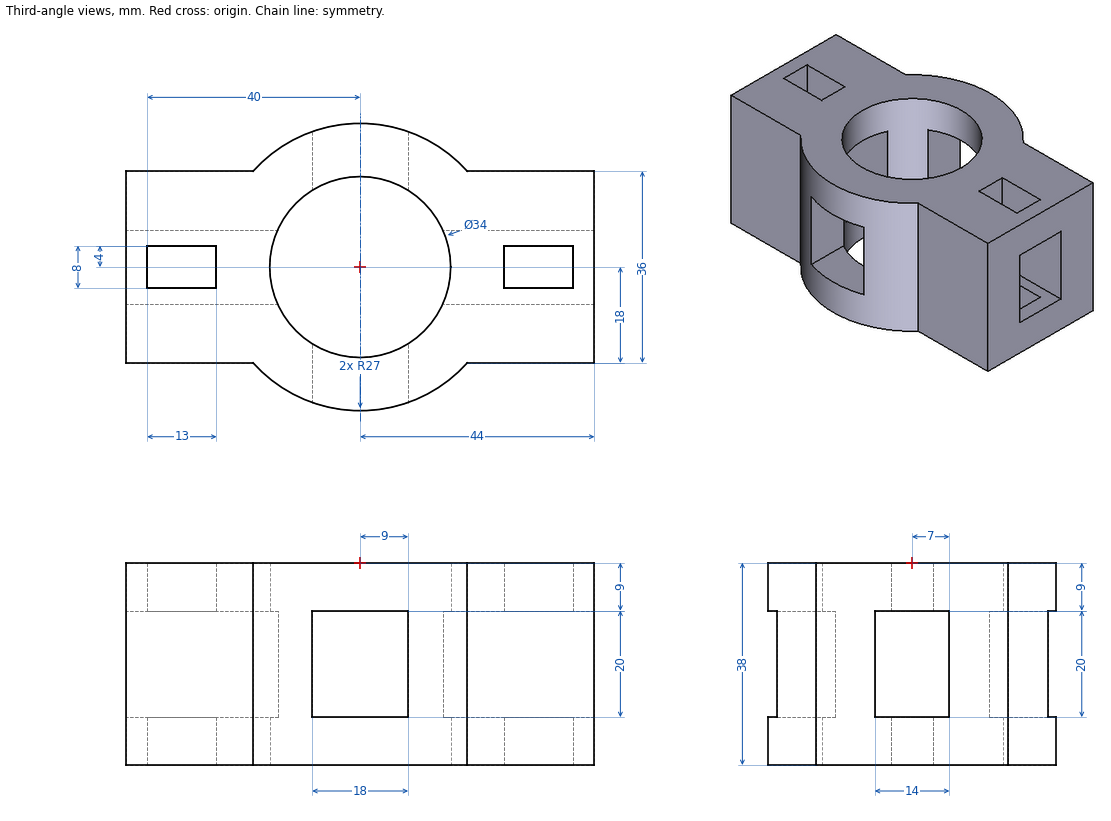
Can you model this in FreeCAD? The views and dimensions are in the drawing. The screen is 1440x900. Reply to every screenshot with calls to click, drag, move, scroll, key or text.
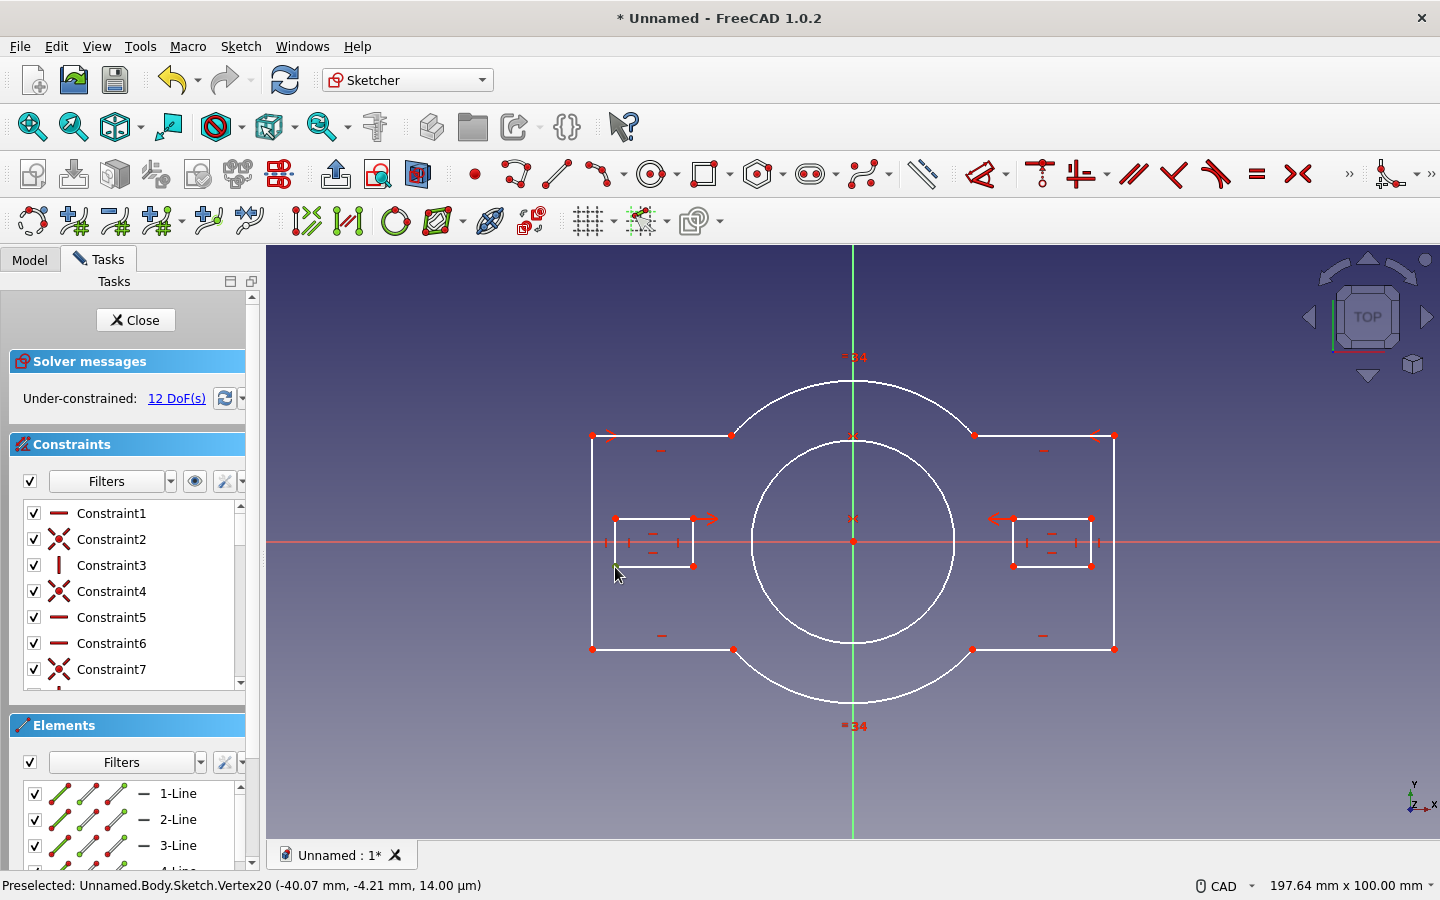
click(1091, 567)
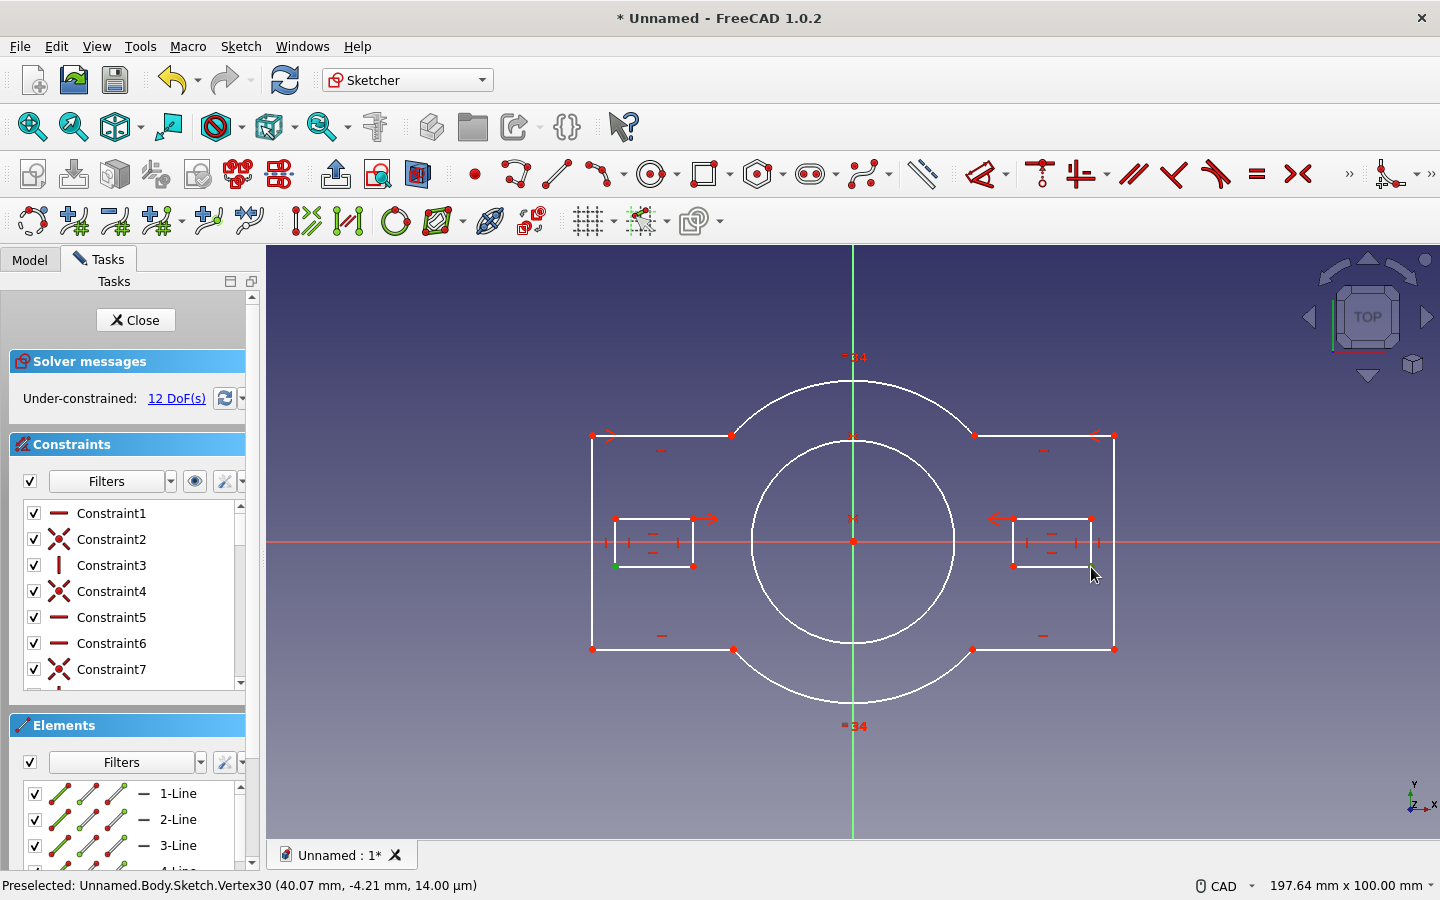
click(853, 773)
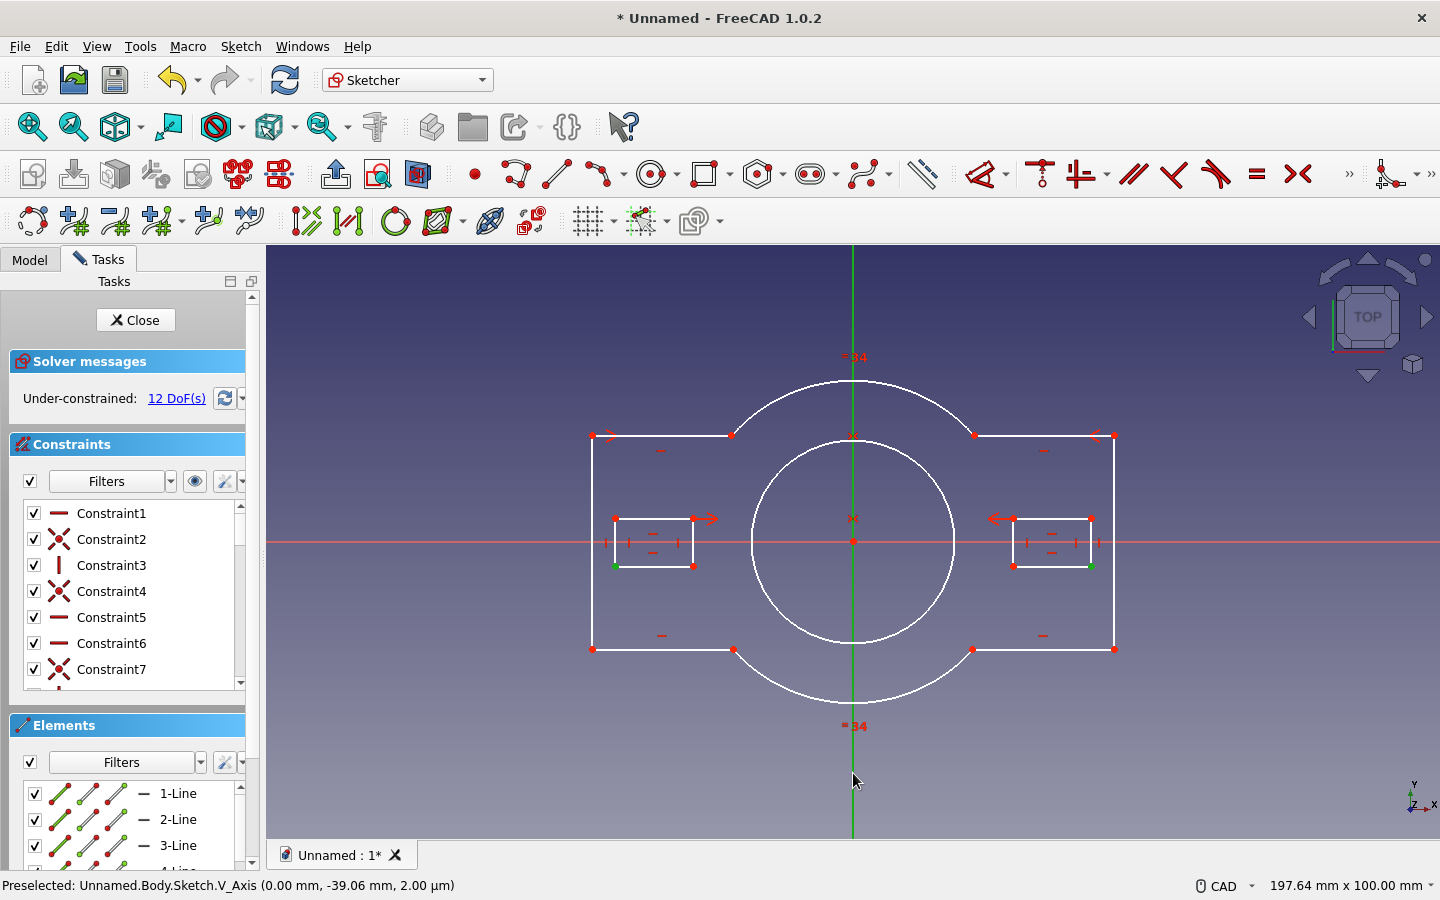
click(1298, 174)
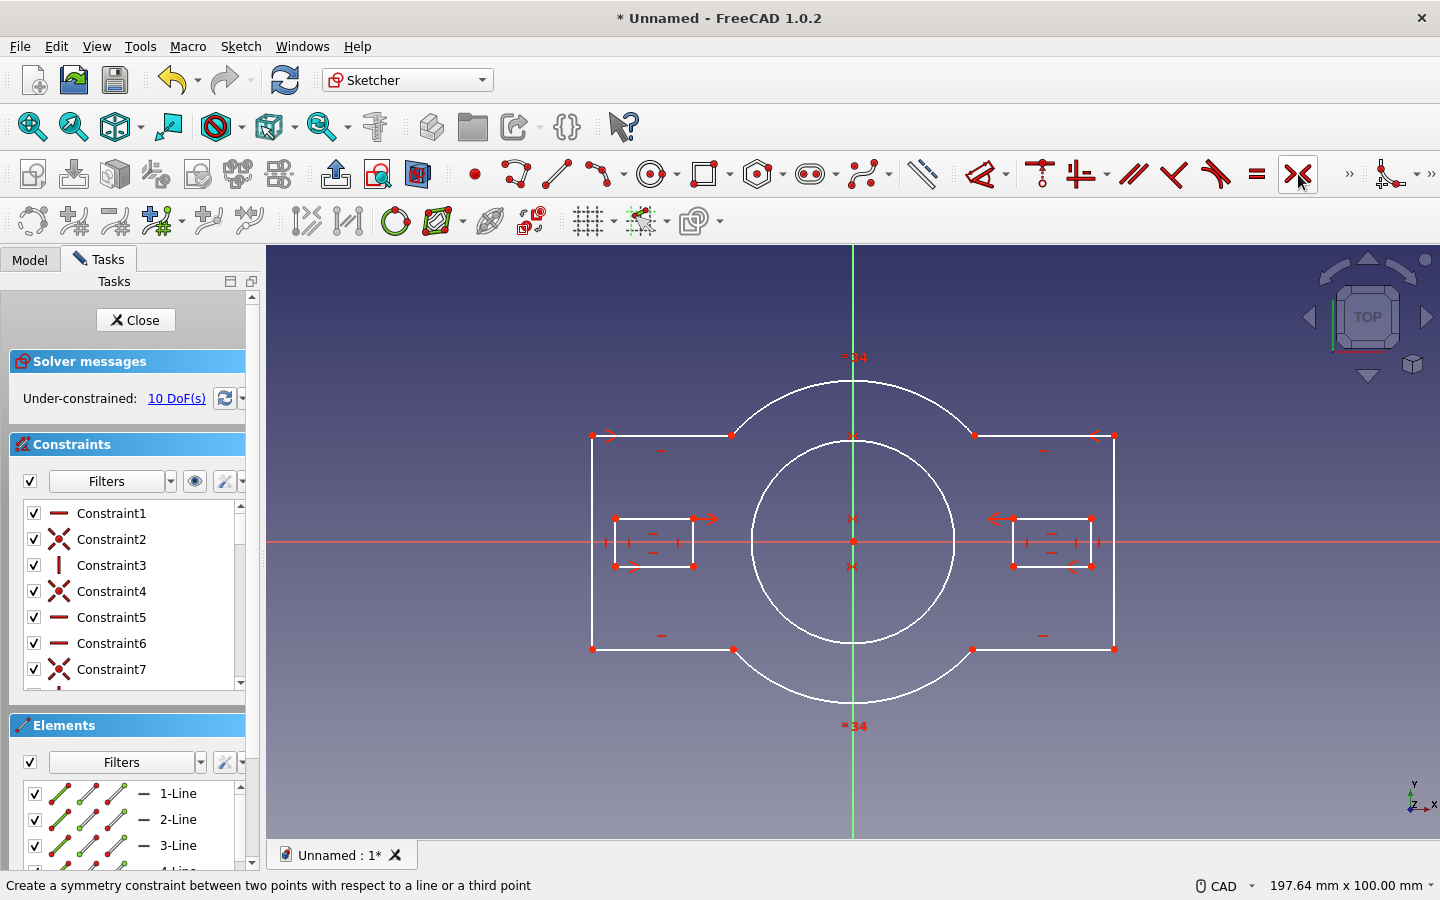
click(980, 174)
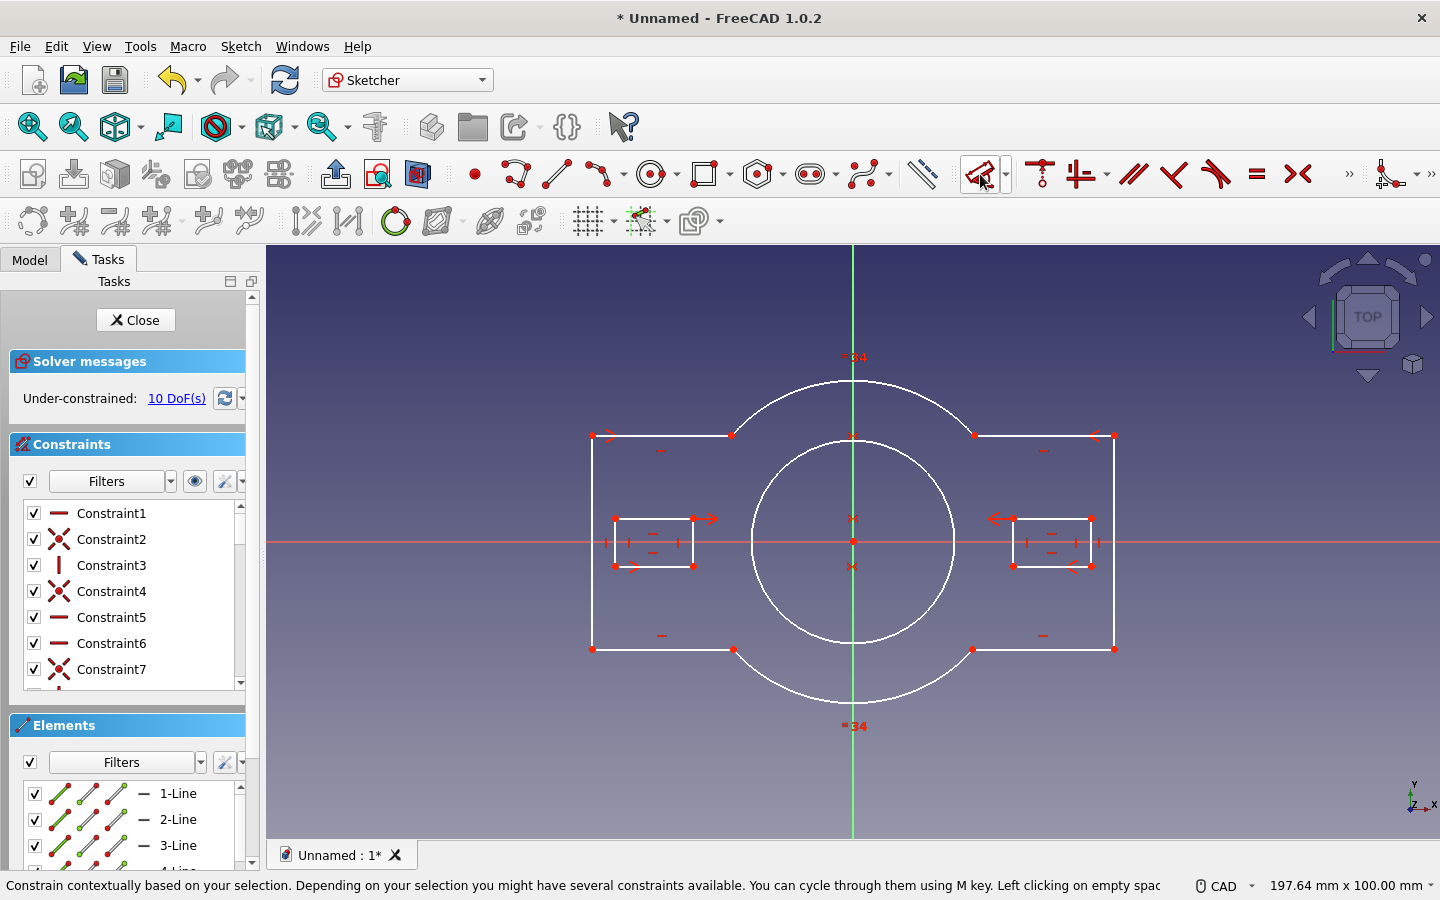
click(907, 390)
click(918, 360)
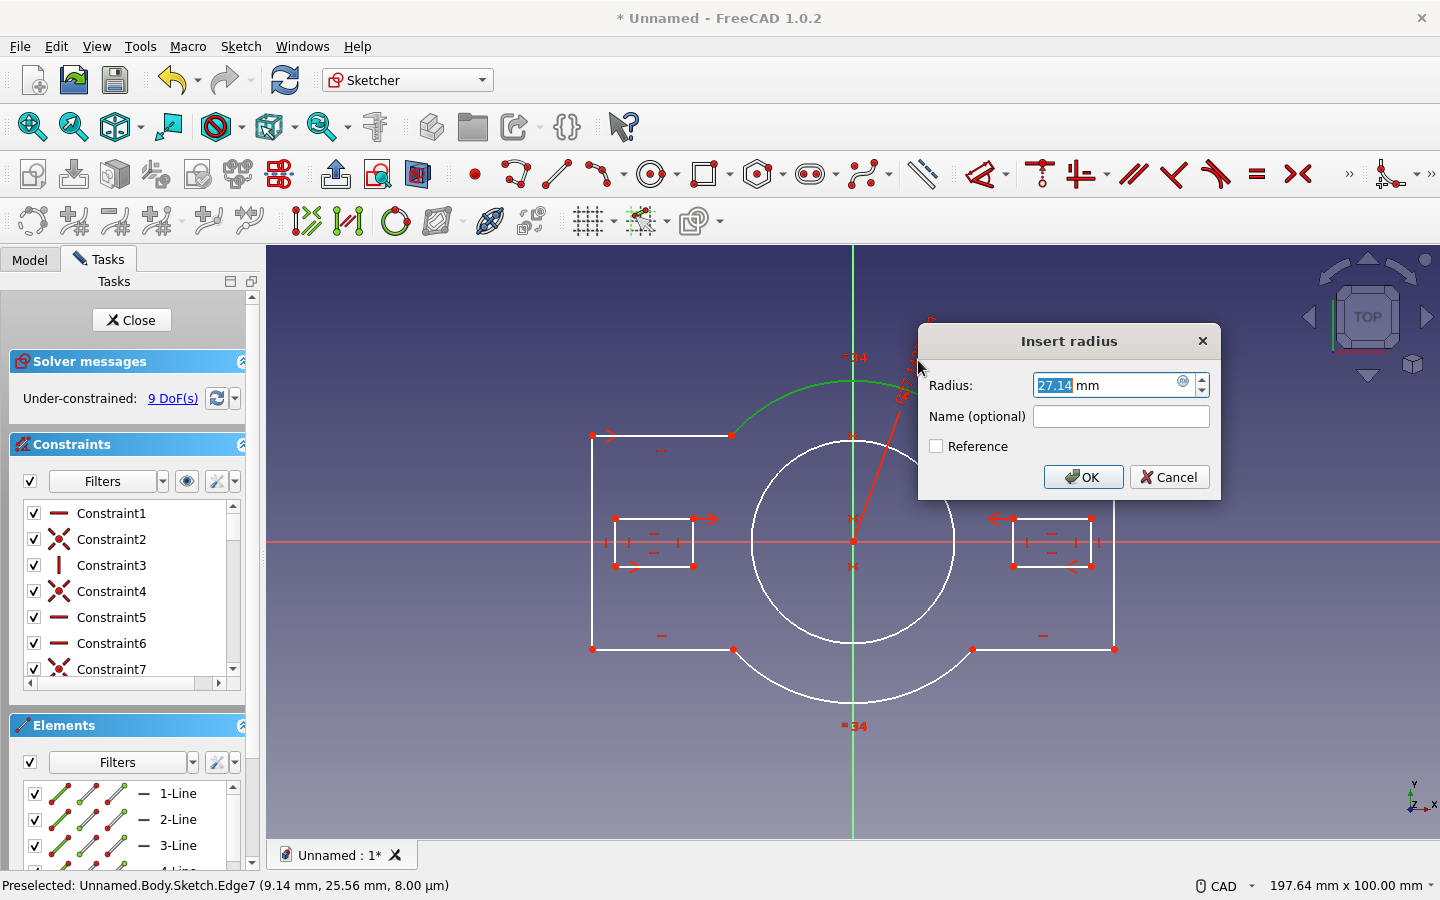
text(27)
key(Return)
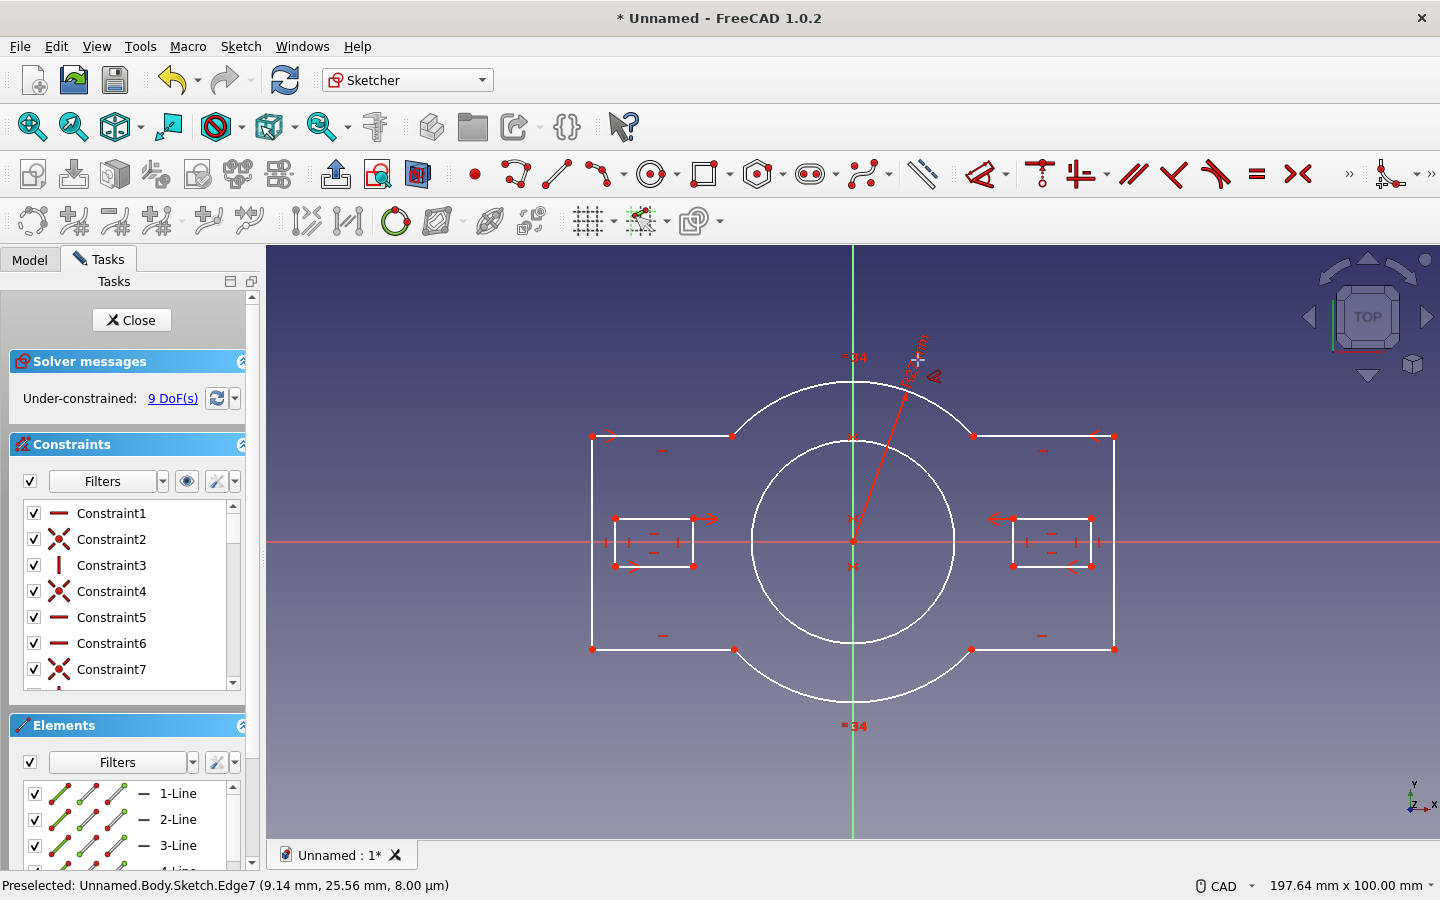
click(925, 470)
click(948, 447)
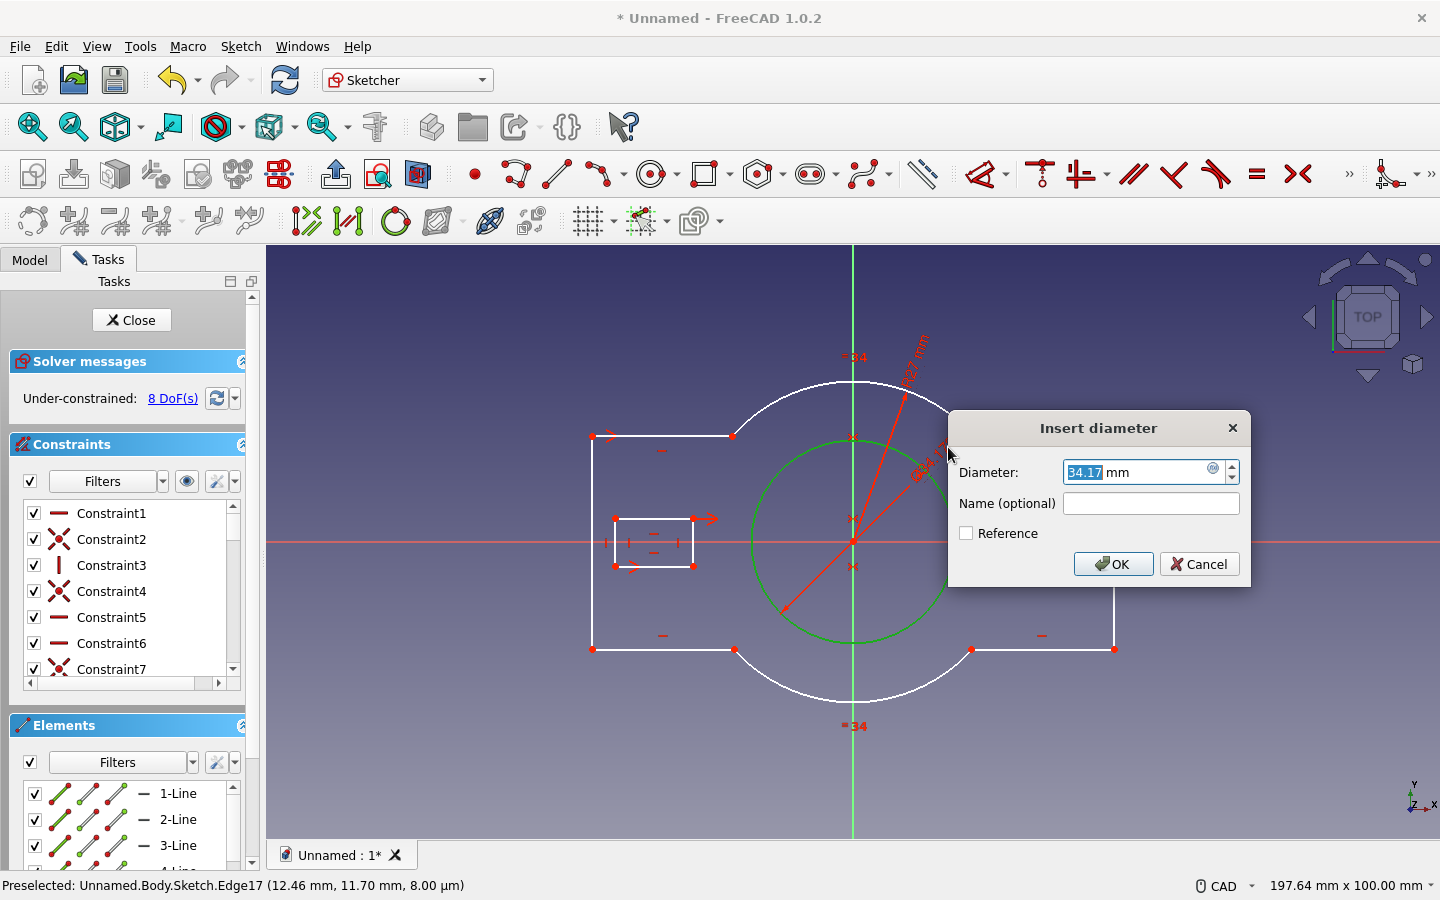
text(34)
key(Return)